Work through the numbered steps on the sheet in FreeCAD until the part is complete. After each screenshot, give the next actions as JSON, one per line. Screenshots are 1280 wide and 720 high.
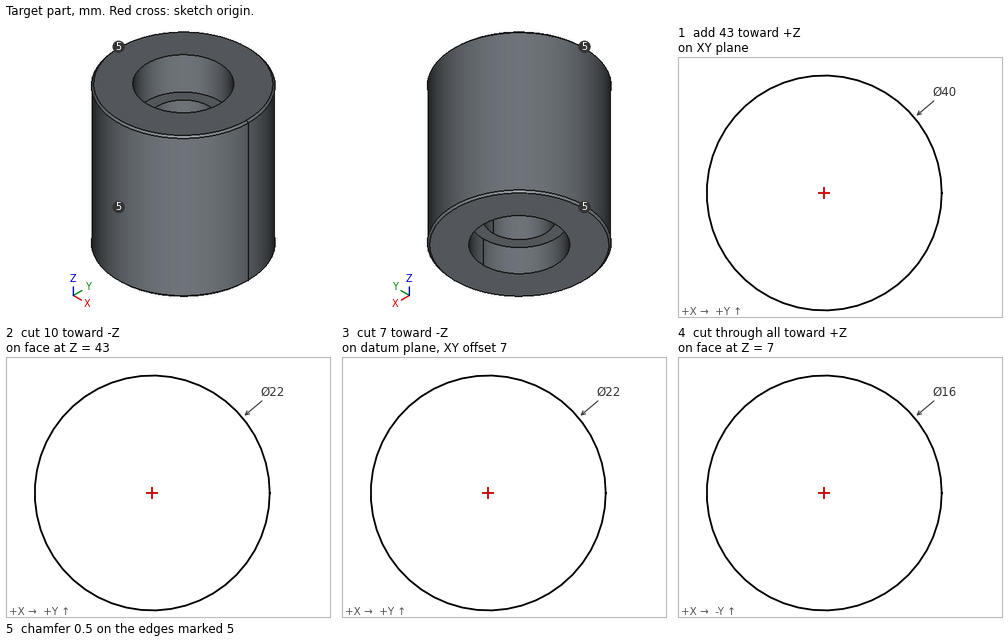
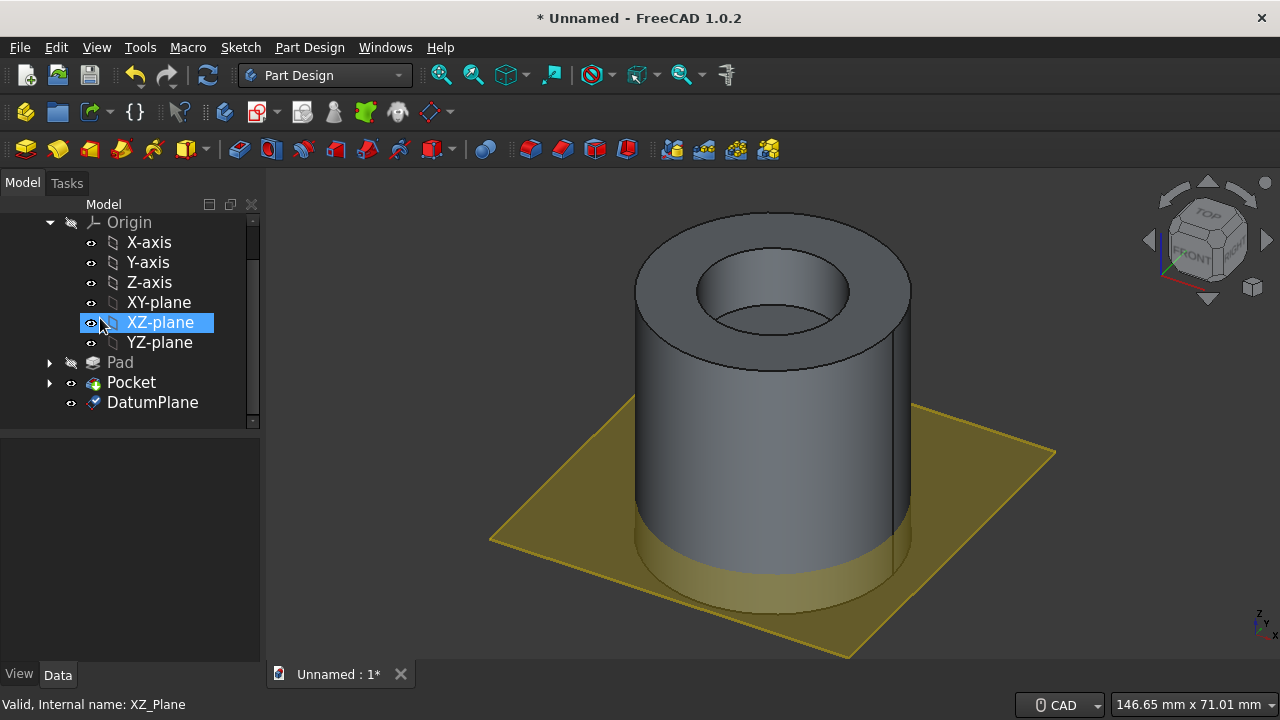
{"action": "left_click", "coordinate": [116, 403]}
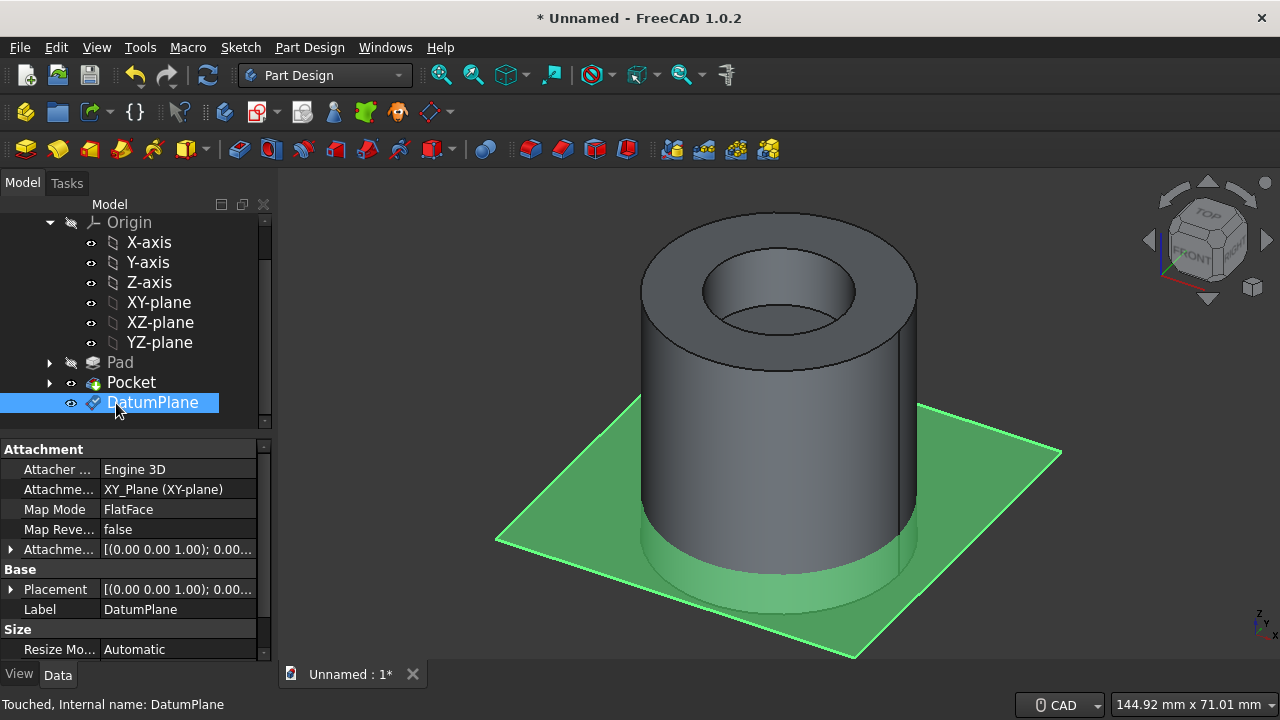
{"action": "left_click", "coordinate": [258, 112]}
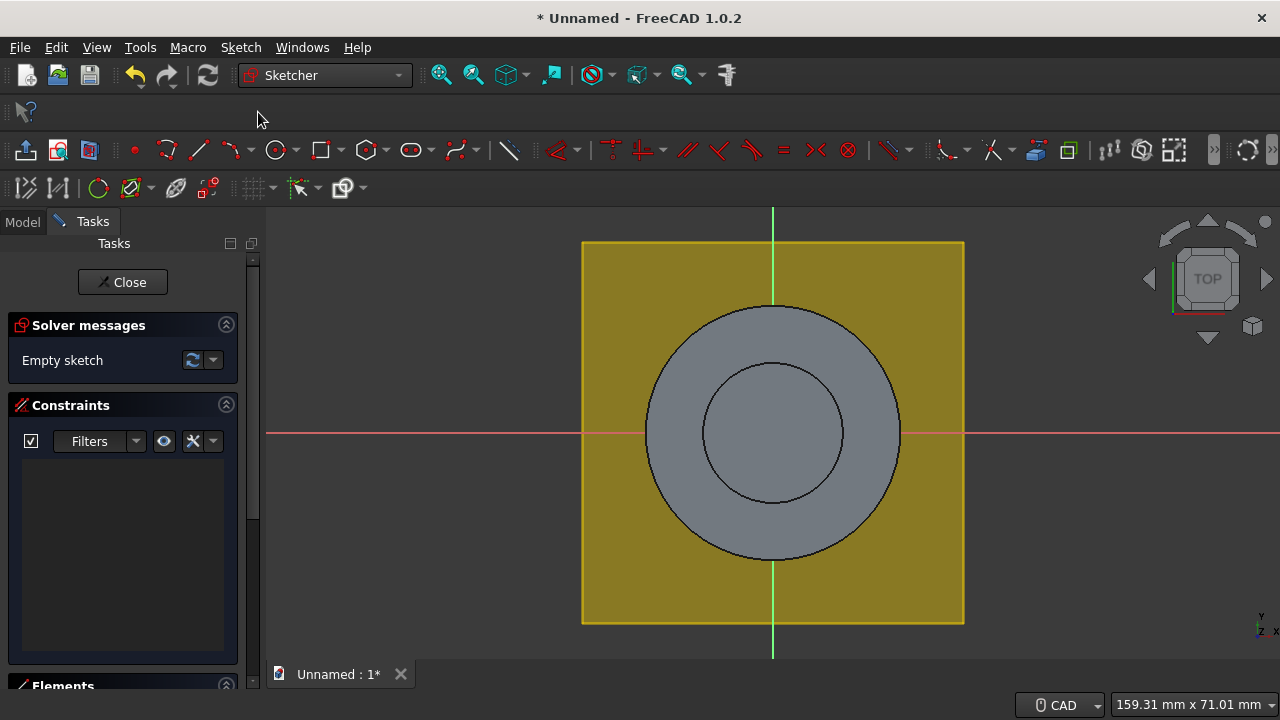
{"action": "left_click", "coordinate": [90, 150]}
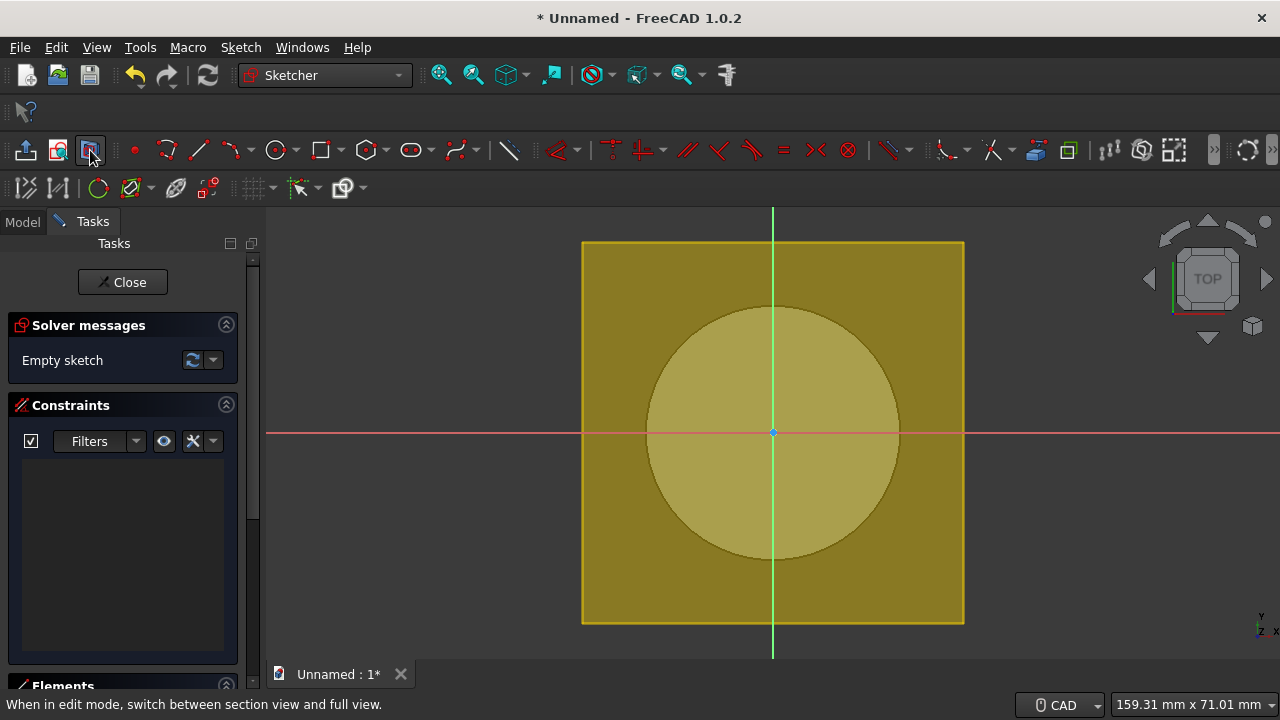
{"action": "scroll", "coordinate": [856, 433], "scroll_direction": "up", "scroll_amount": 3}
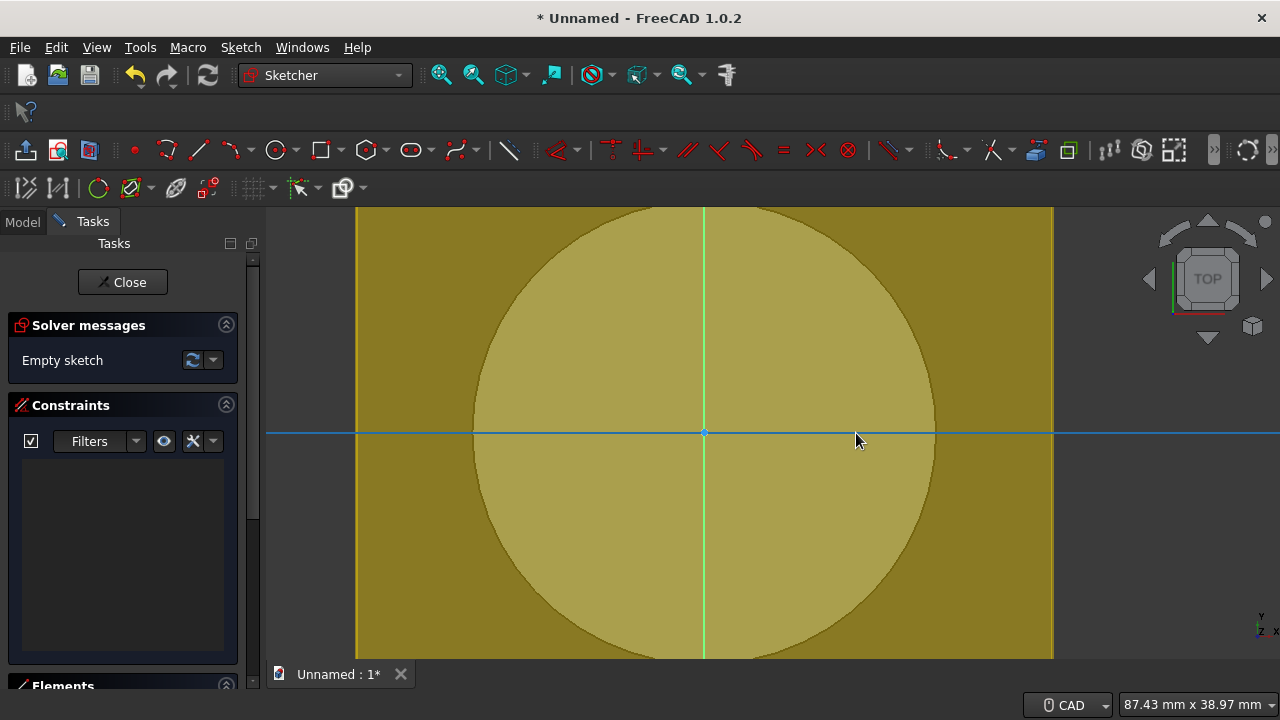
{"action": "left_click", "coordinate": [276, 150]}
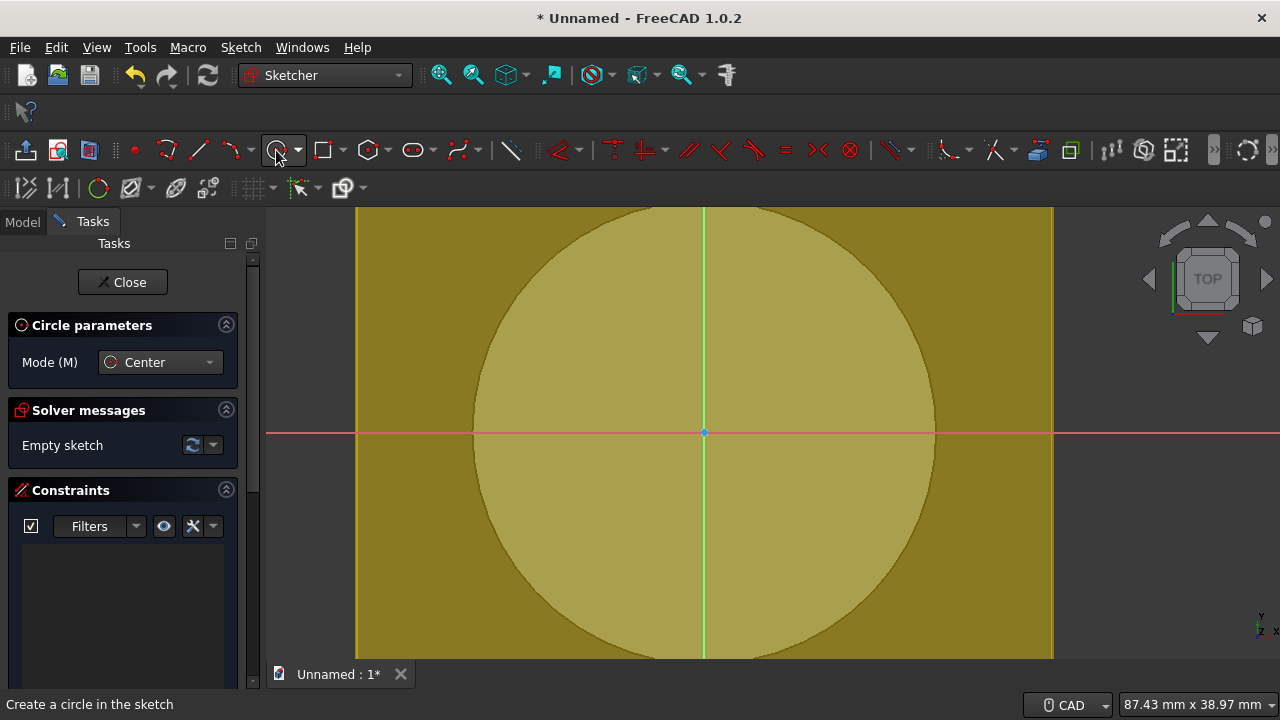
{"action": "left_click", "coordinate": [704, 433]}
{"action": "mouse_move", "coordinate": [794, 342]}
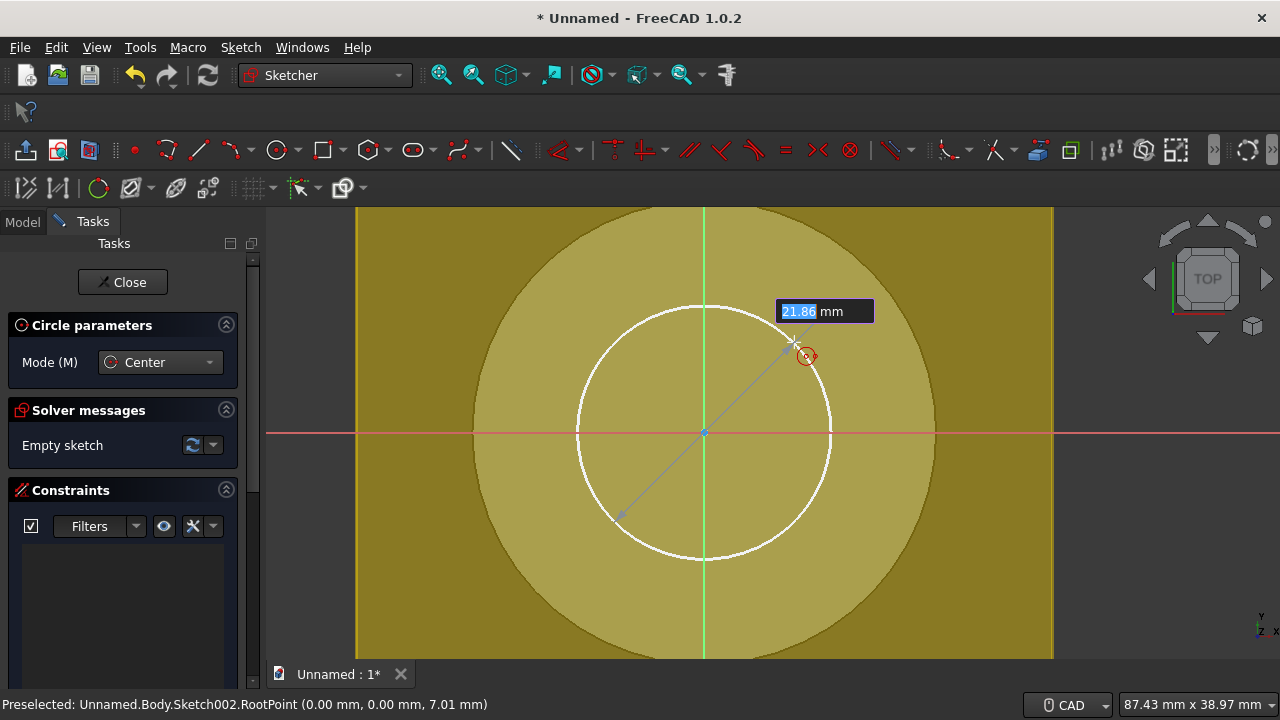
{"action": "type", "text": "22"}
{"action": "key", "text": "Return"}
{"action": "key", "text": "Escape"}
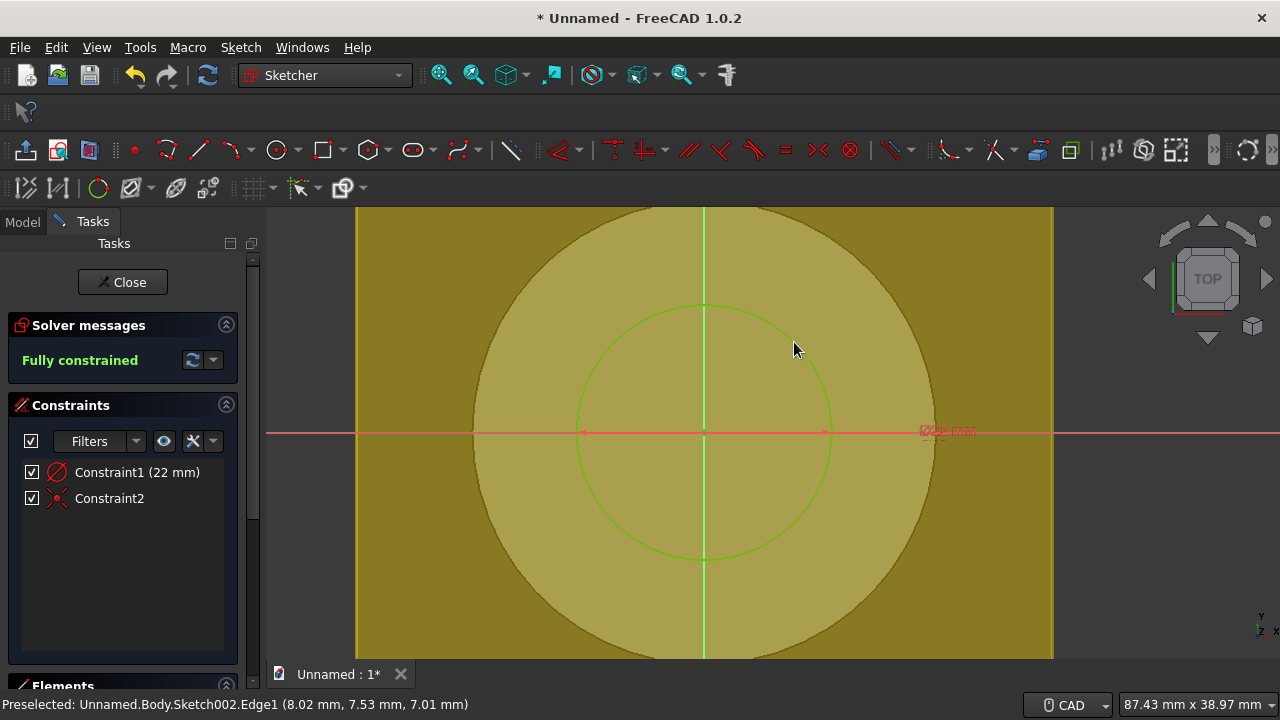
{"action": "left_click", "coordinate": [123, 282]}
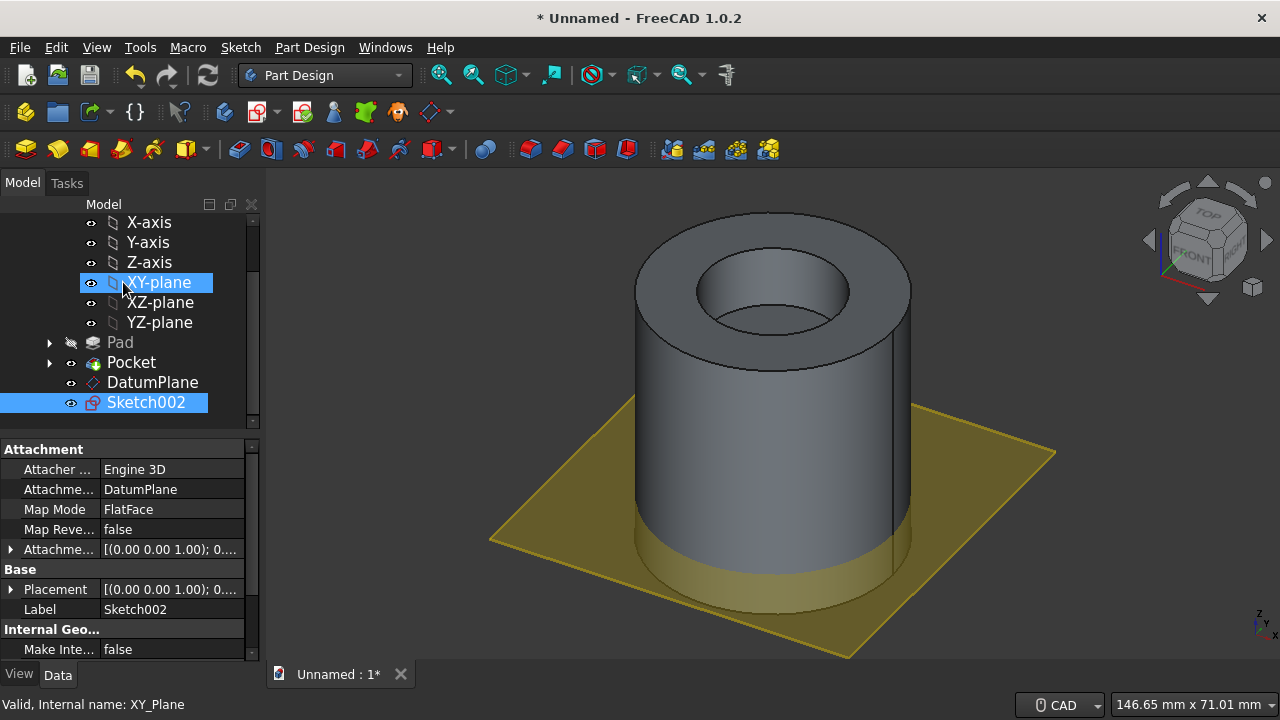
{"action": "left_click", "coordinate": [240, 150]}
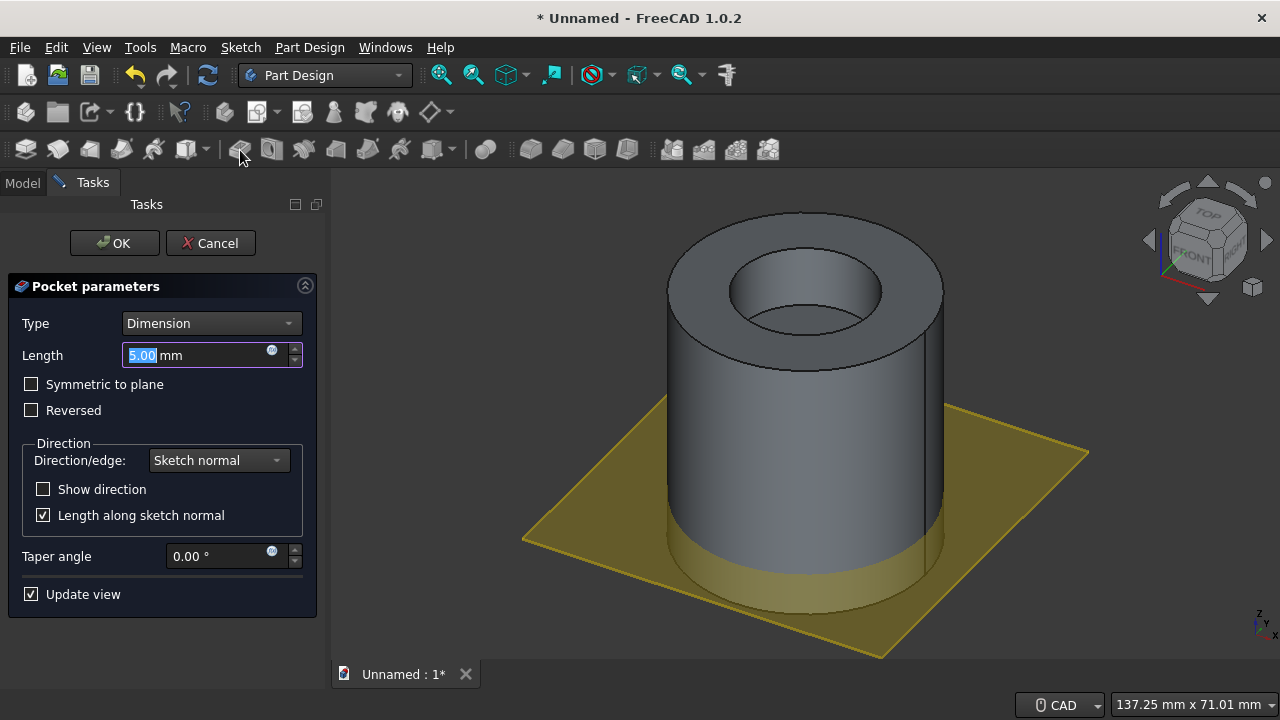
{"action": "type", "text": "7"}
{"action": "key", "text": "Tab"}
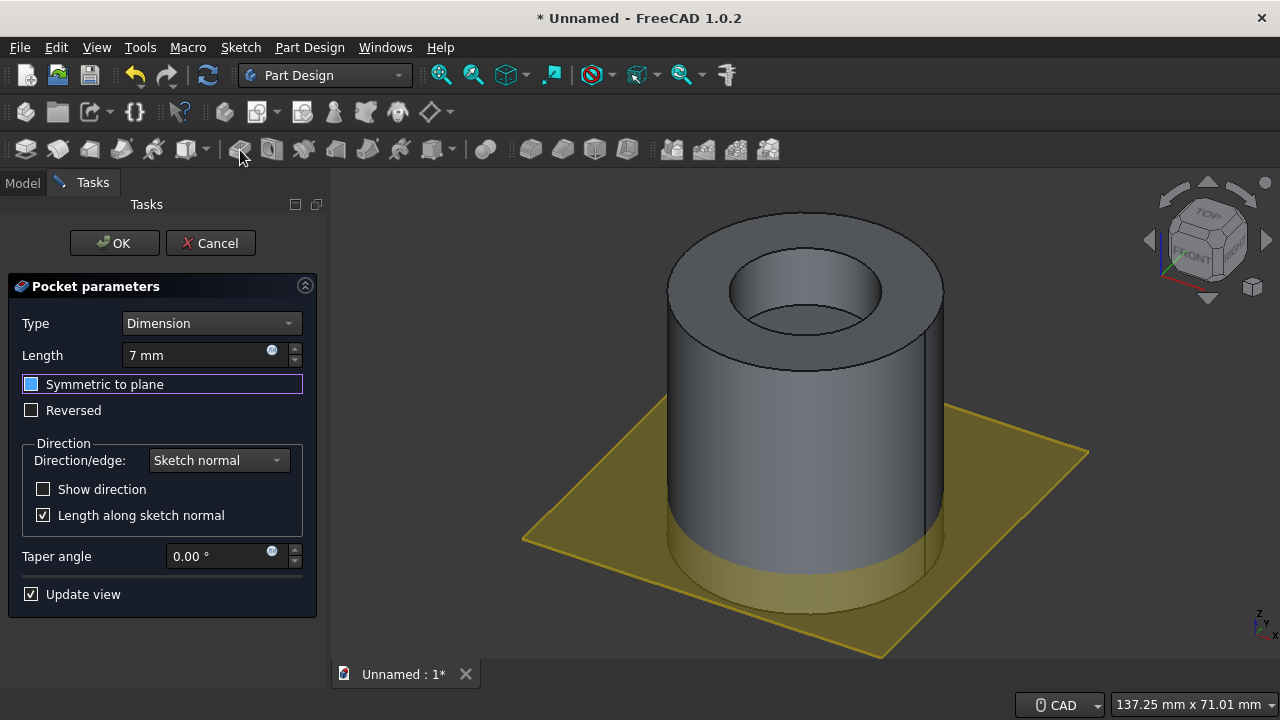
{"action": "left_click", "coordinate": [115, 243]}